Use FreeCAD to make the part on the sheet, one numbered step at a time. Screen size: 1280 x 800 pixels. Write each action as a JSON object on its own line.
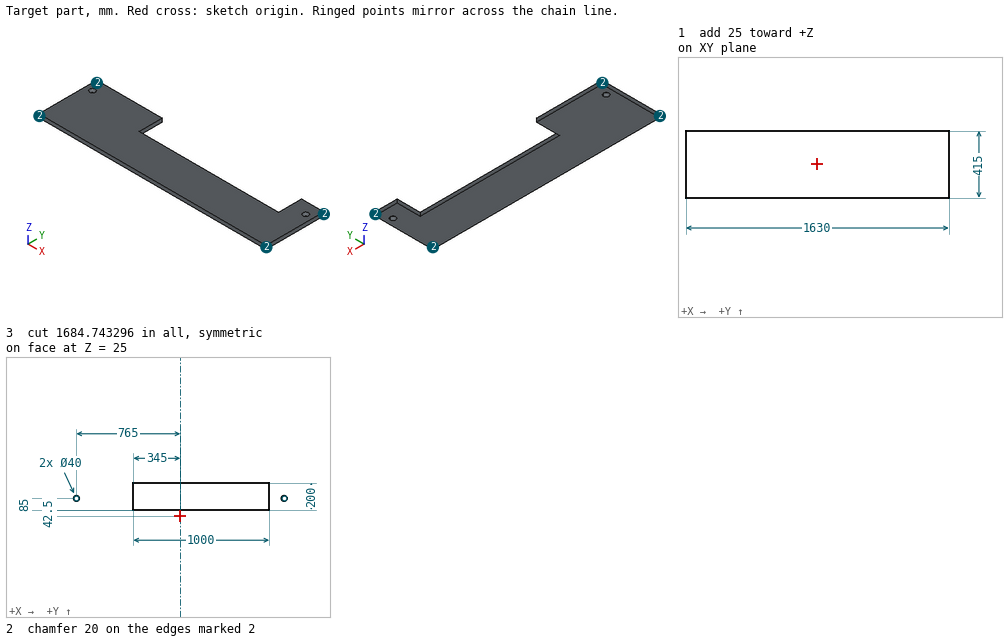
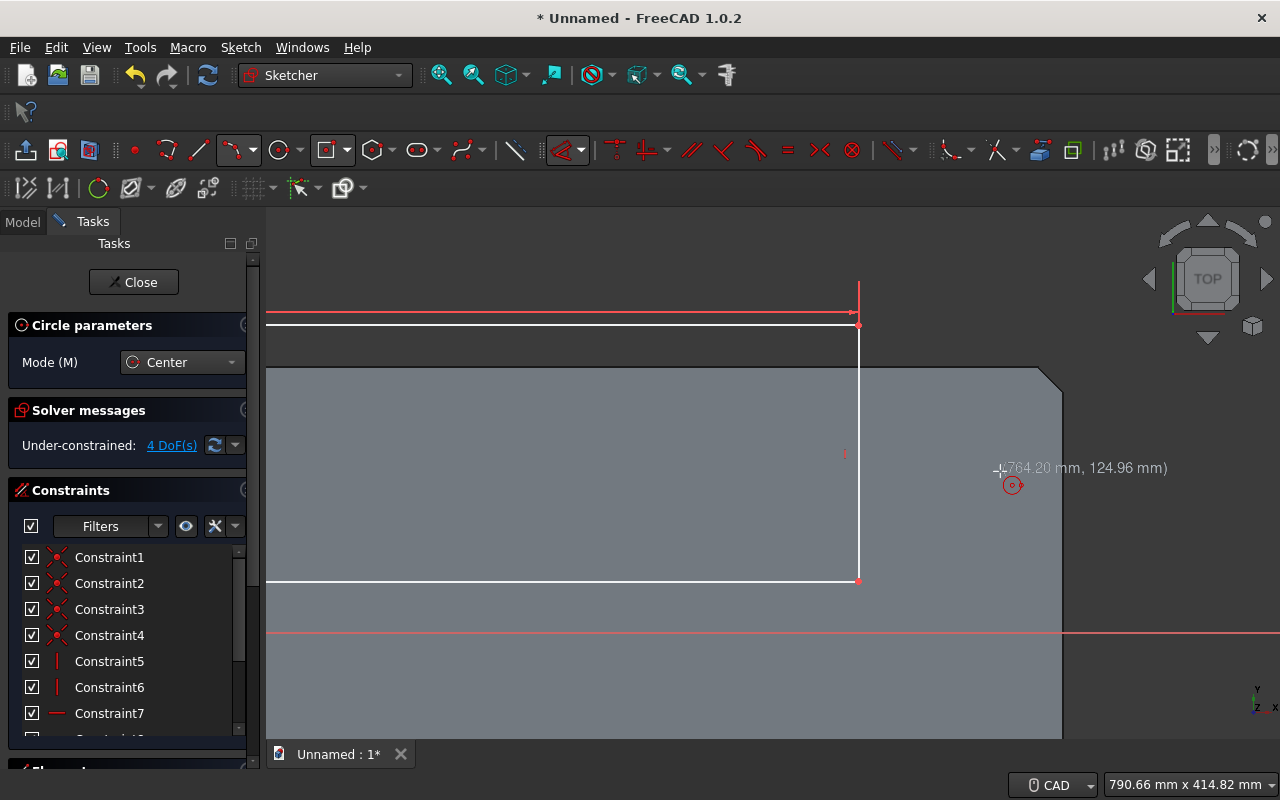
{"action": "scroll", "coordinate": [1000, 471], "scroll_direction": "down", "scroll_amount": 6}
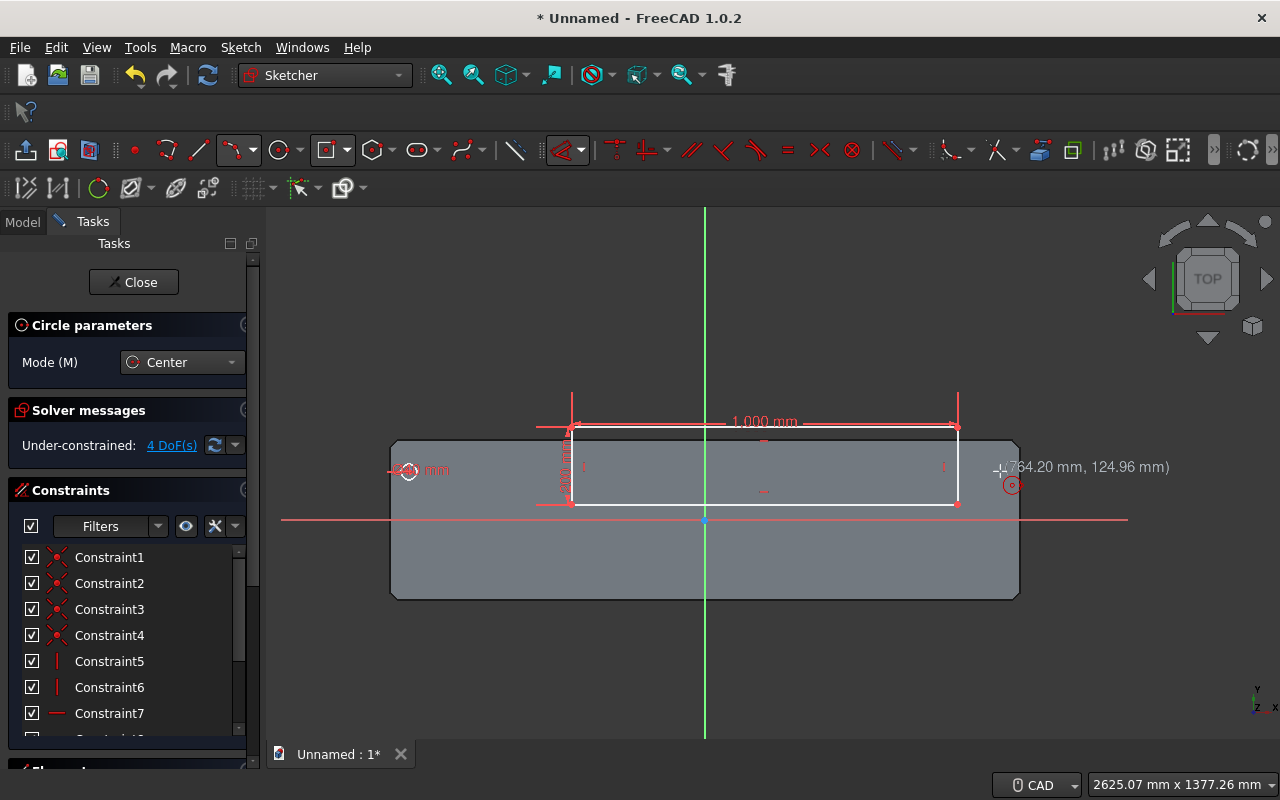
{"action": "left_click", "coordinate": [1000, 471]}
{"action": "mouse_move", "coordinate": [1006, 466]}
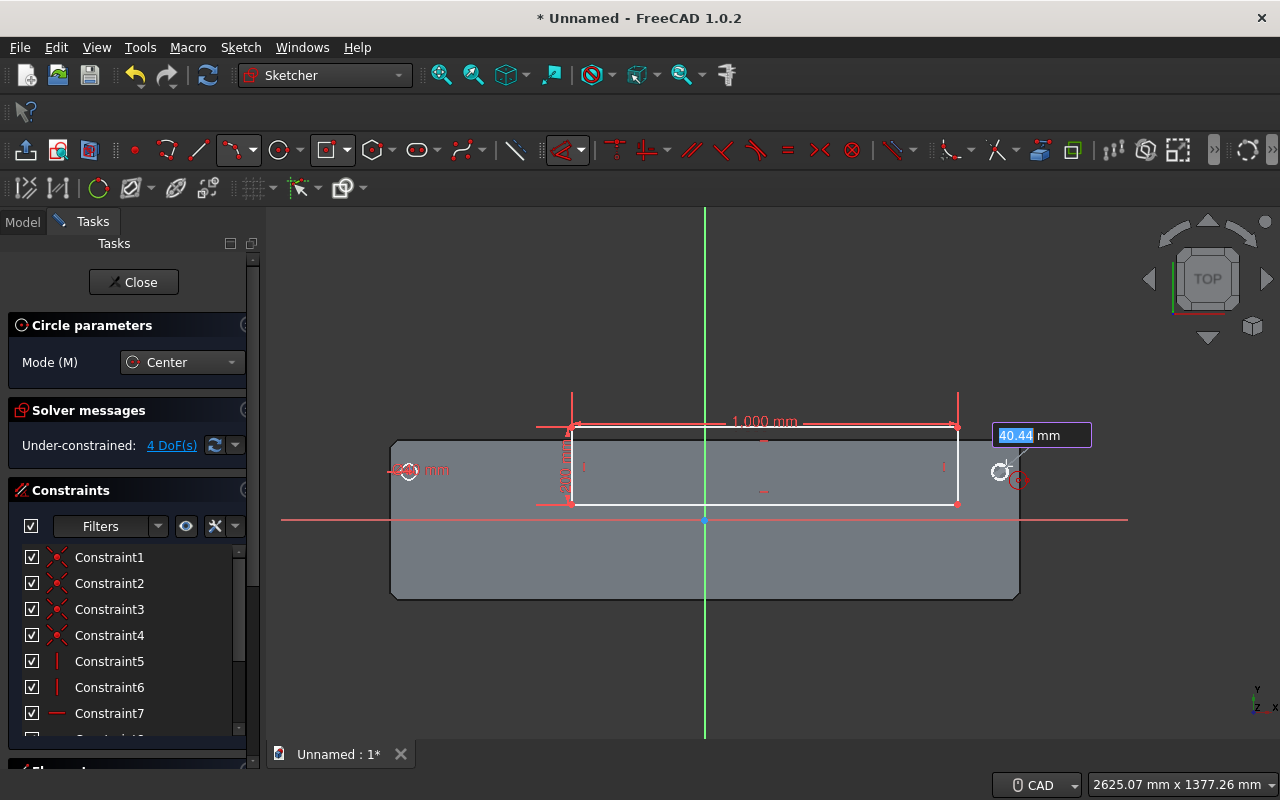
{"action": "type", "text": "40"}
{"action": "key", "text": "Return"}
{"action": "key", "text": "Escape"}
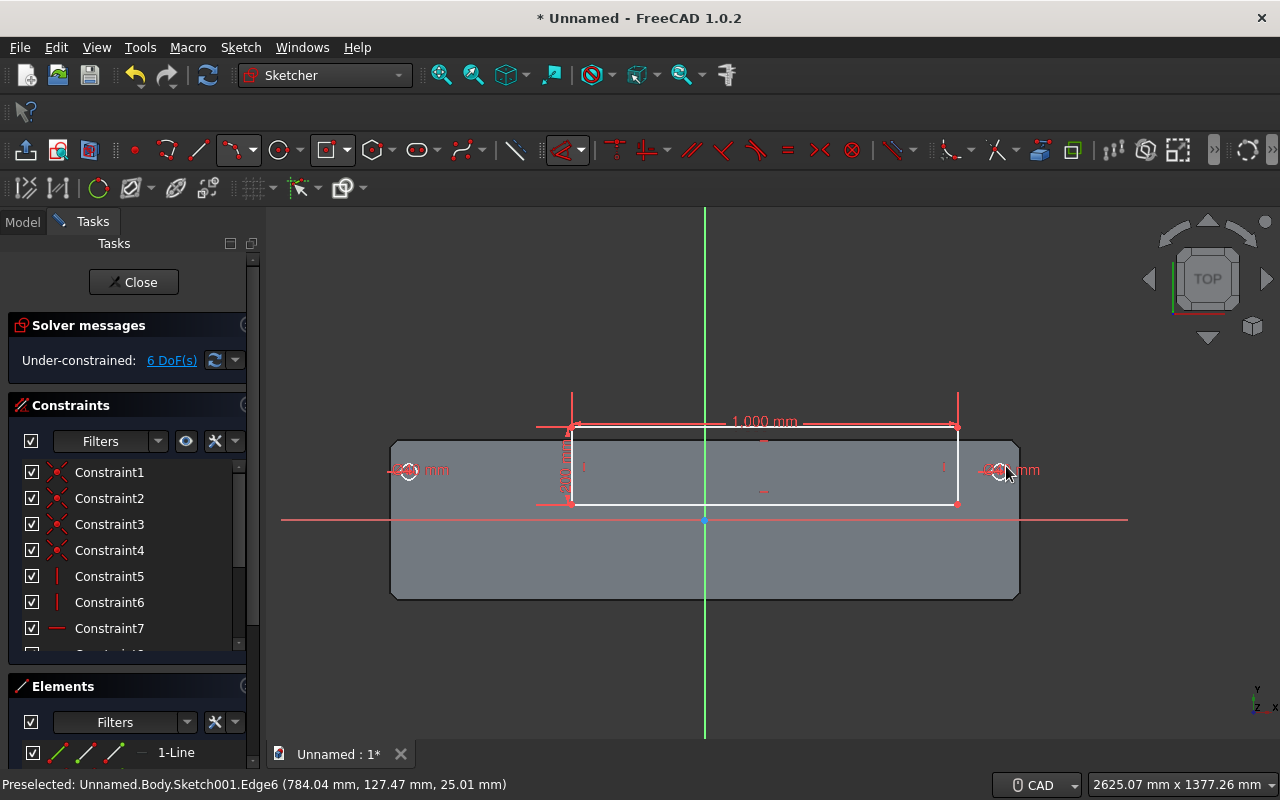
{"action": "left_click", "coordinate": [409, 472]}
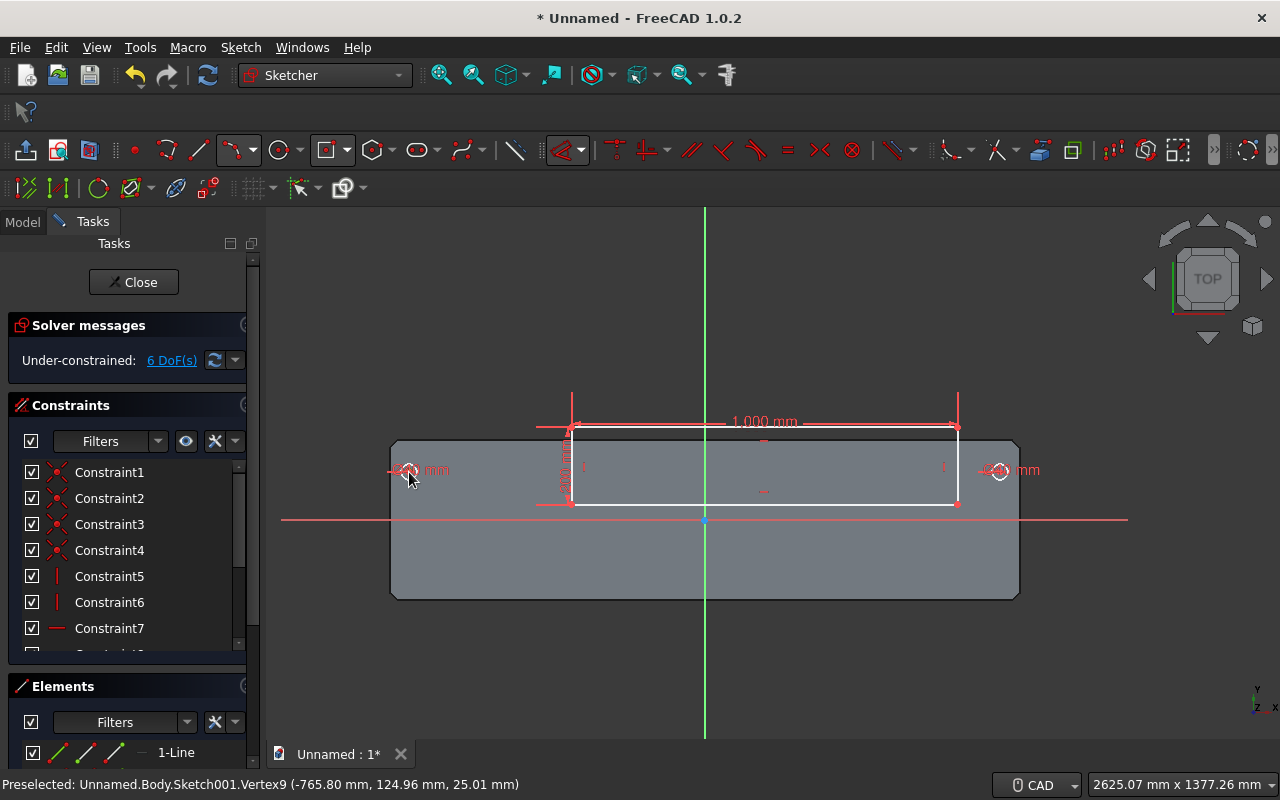
{"action": "left_click", "coordinate": [1000, 472]}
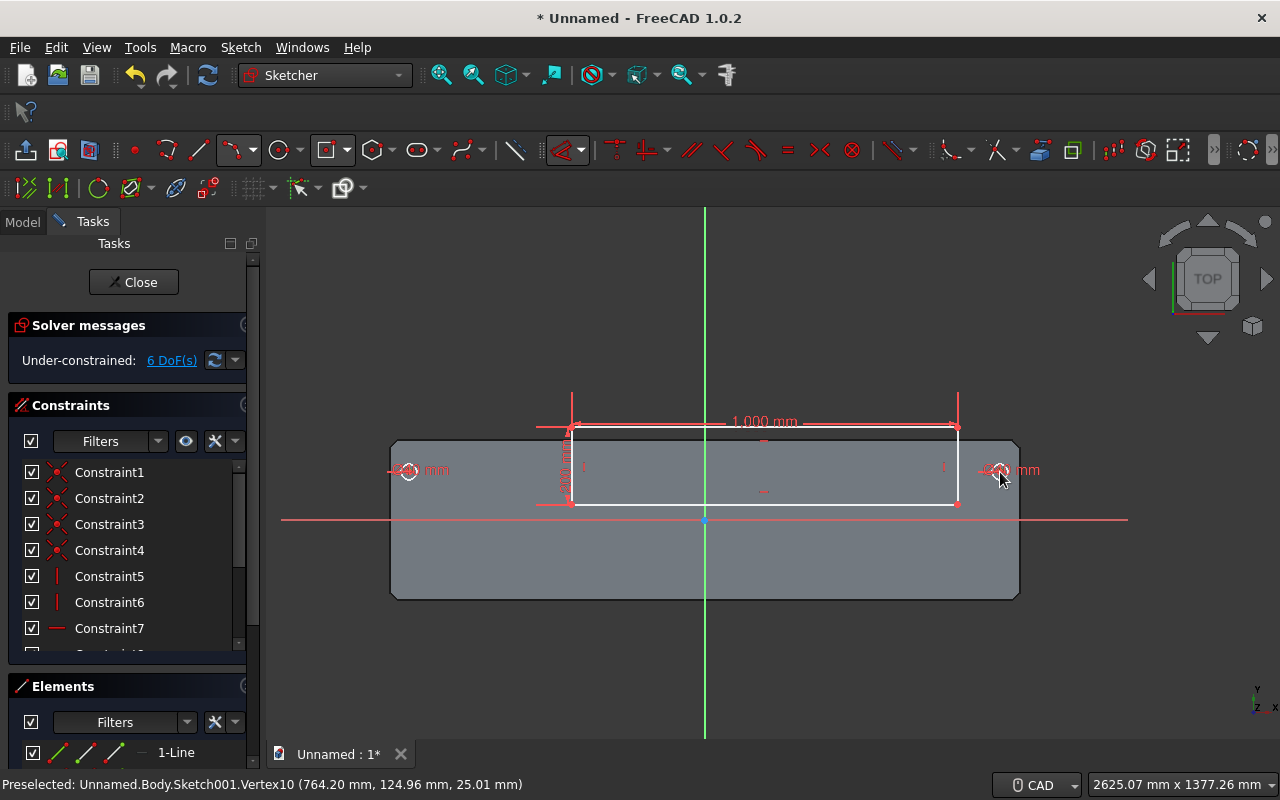
{"action": "left_click", "coordinate": [705, 677]}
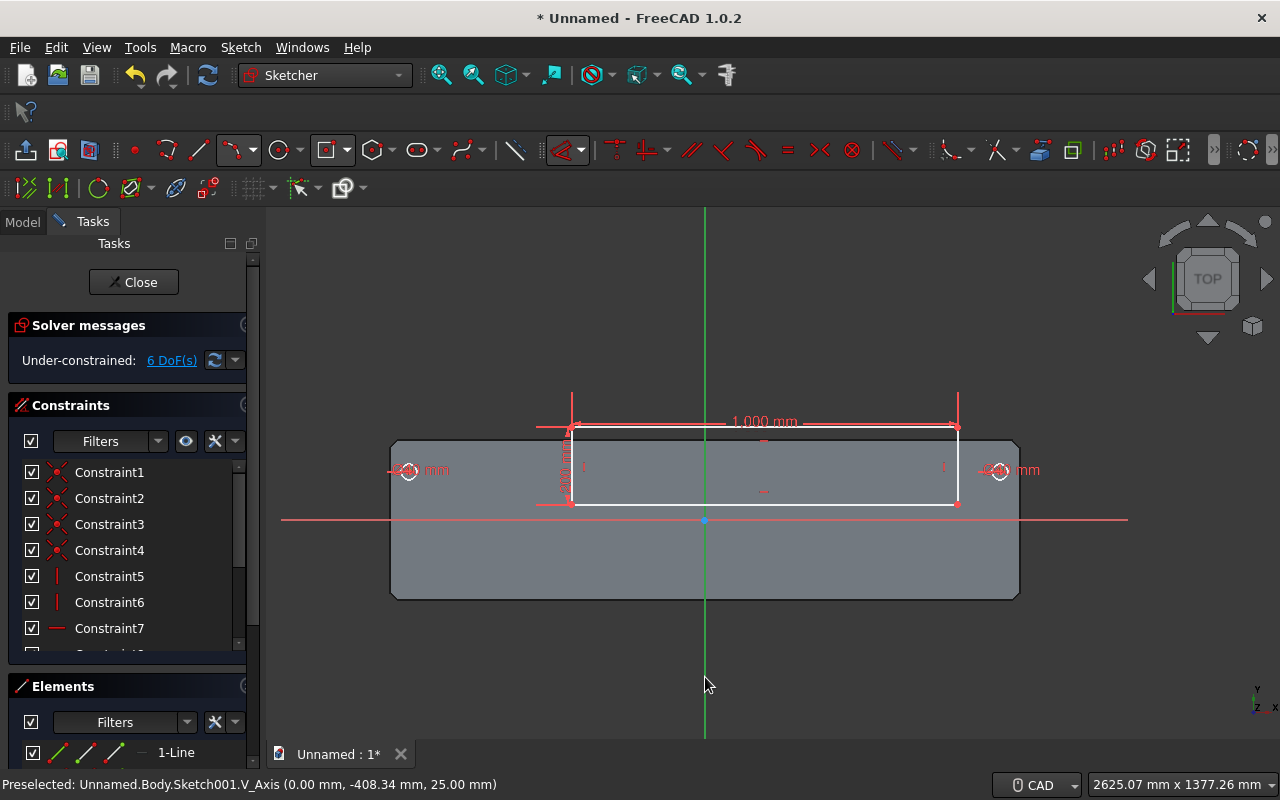
{"action": "left_click", "coordinate": [820, 150]}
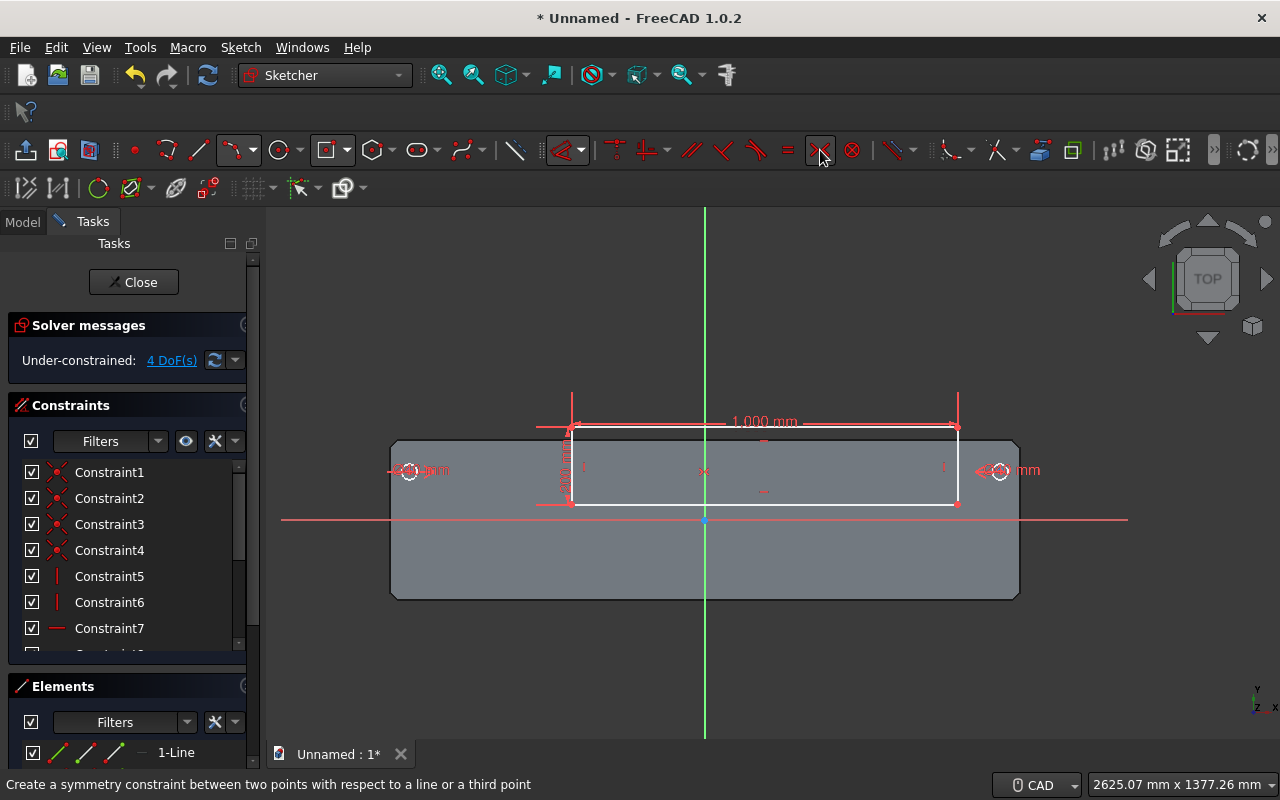
{"action": "left_click", "coordinate": [562, 150]}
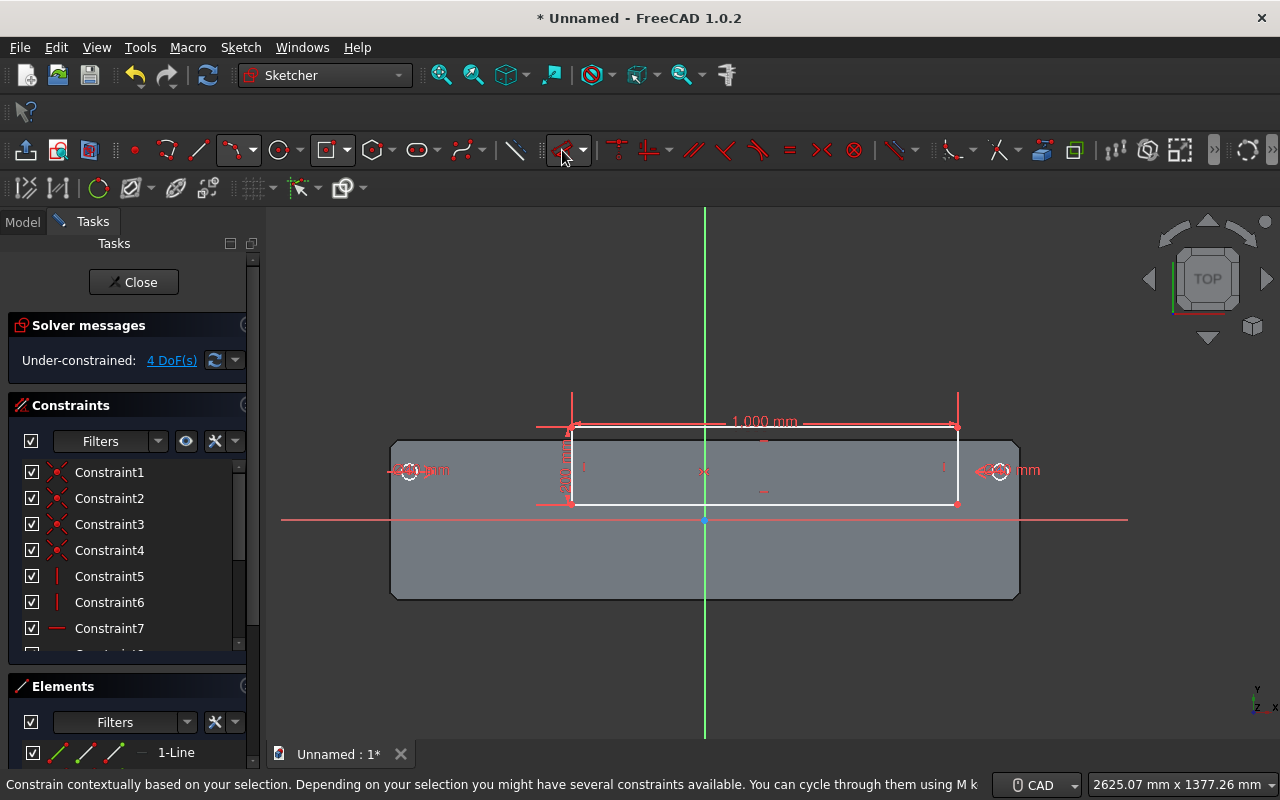
{"action": "left_click", "coordinate": [409, 472]}
{"action": "left_click", "coordinate": [557, 554]}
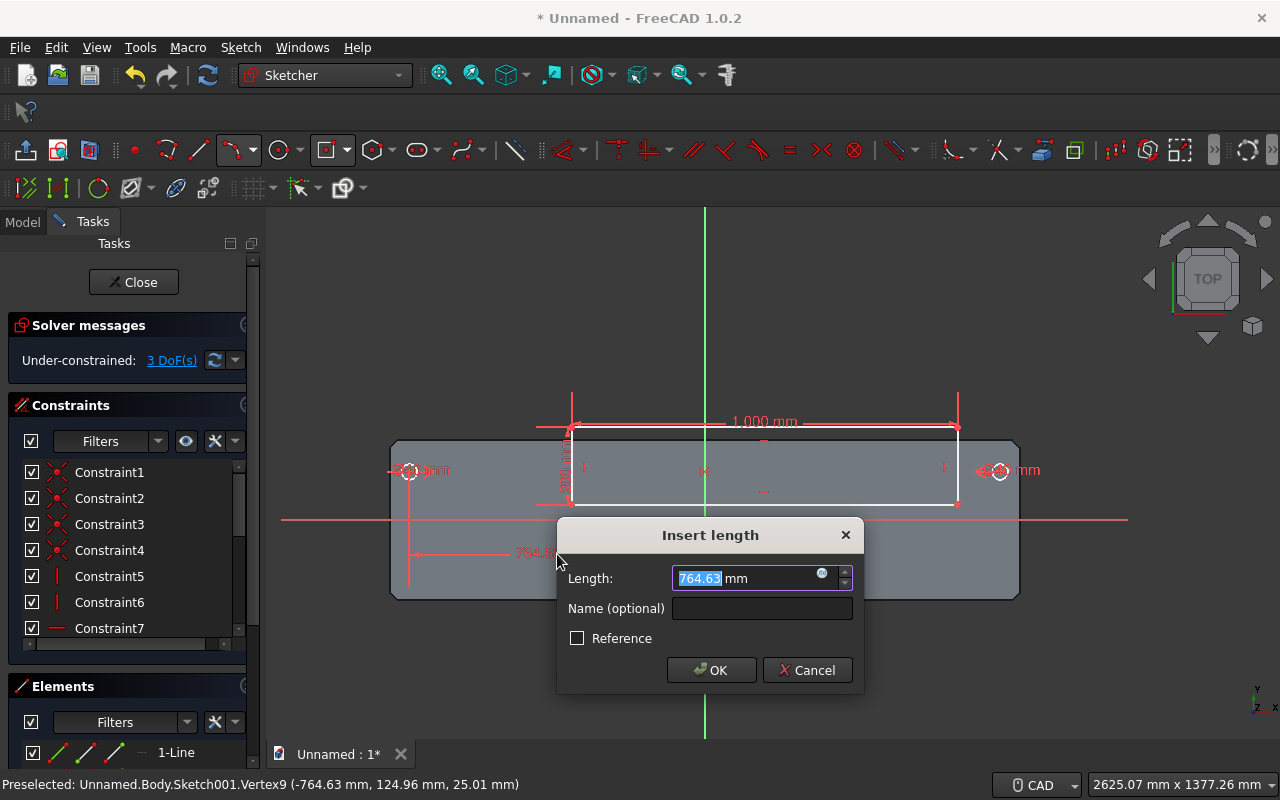
{"action": "type", "text": "765"}
{"action": "key", "text": "Return"}